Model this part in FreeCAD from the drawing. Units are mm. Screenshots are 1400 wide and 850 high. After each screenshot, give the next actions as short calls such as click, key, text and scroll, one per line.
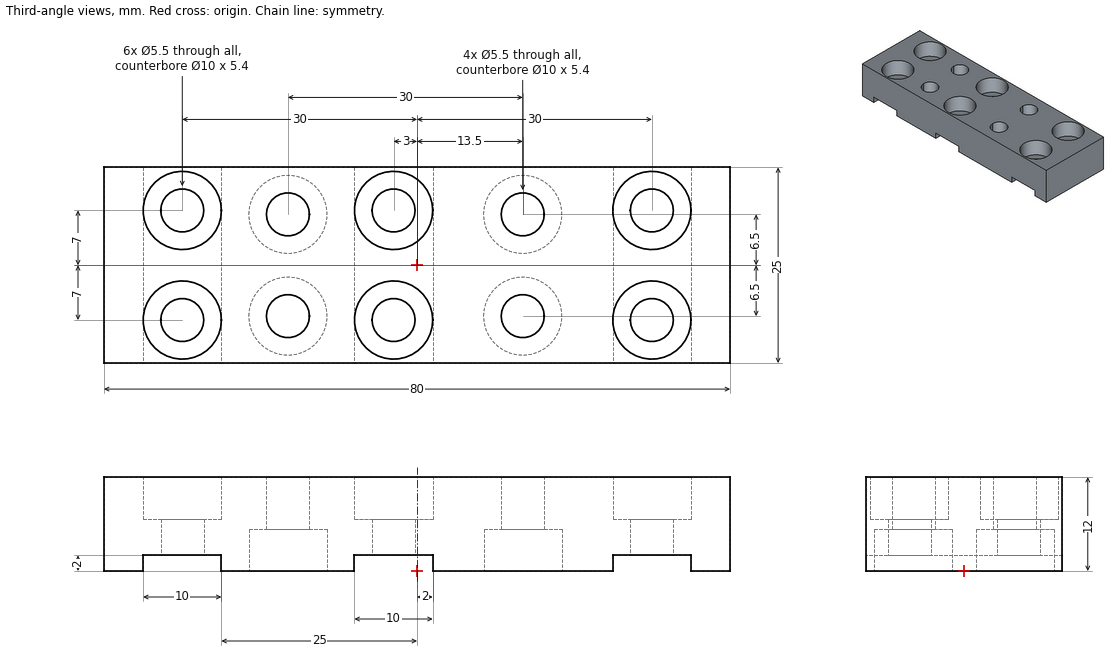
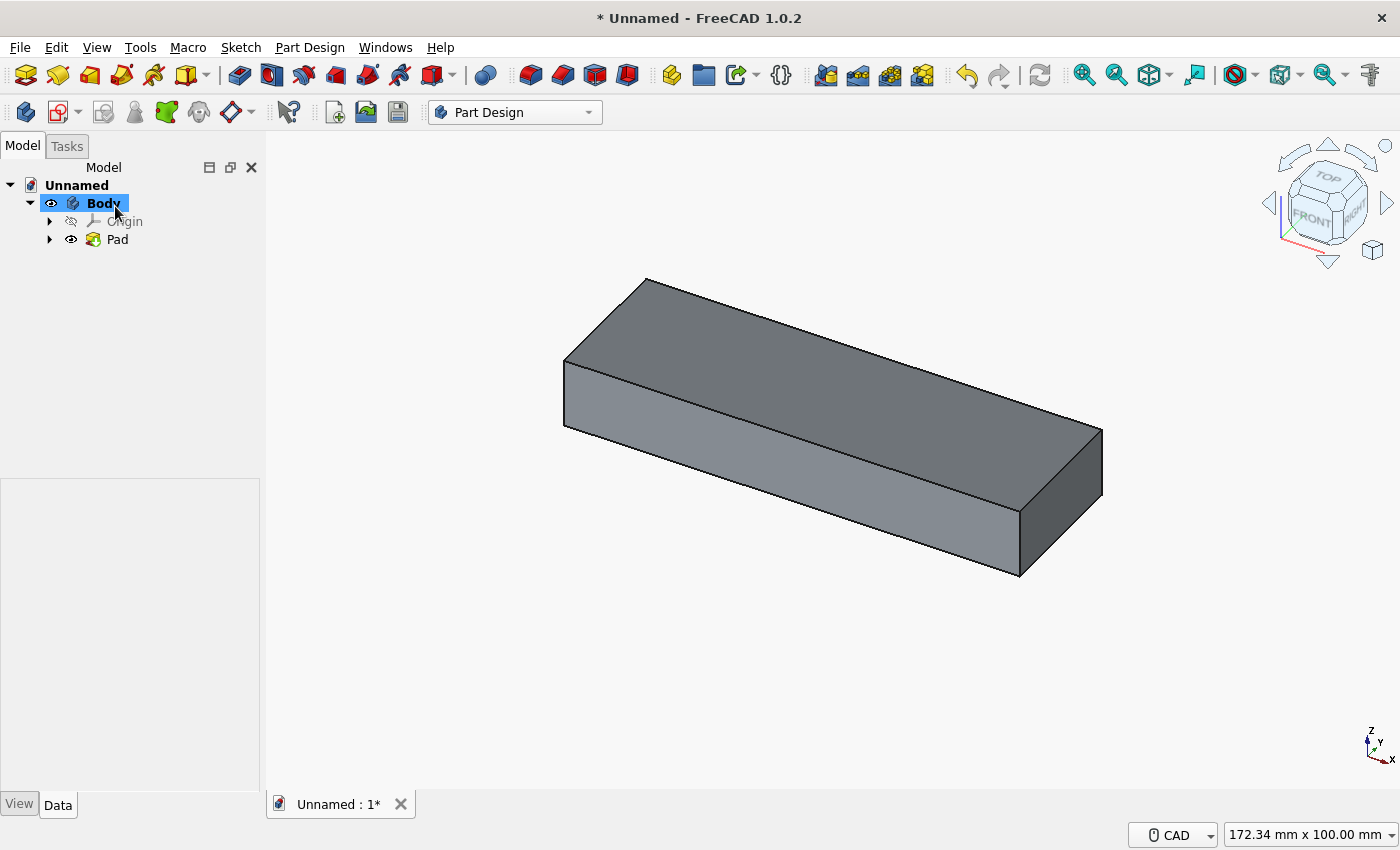
key(4)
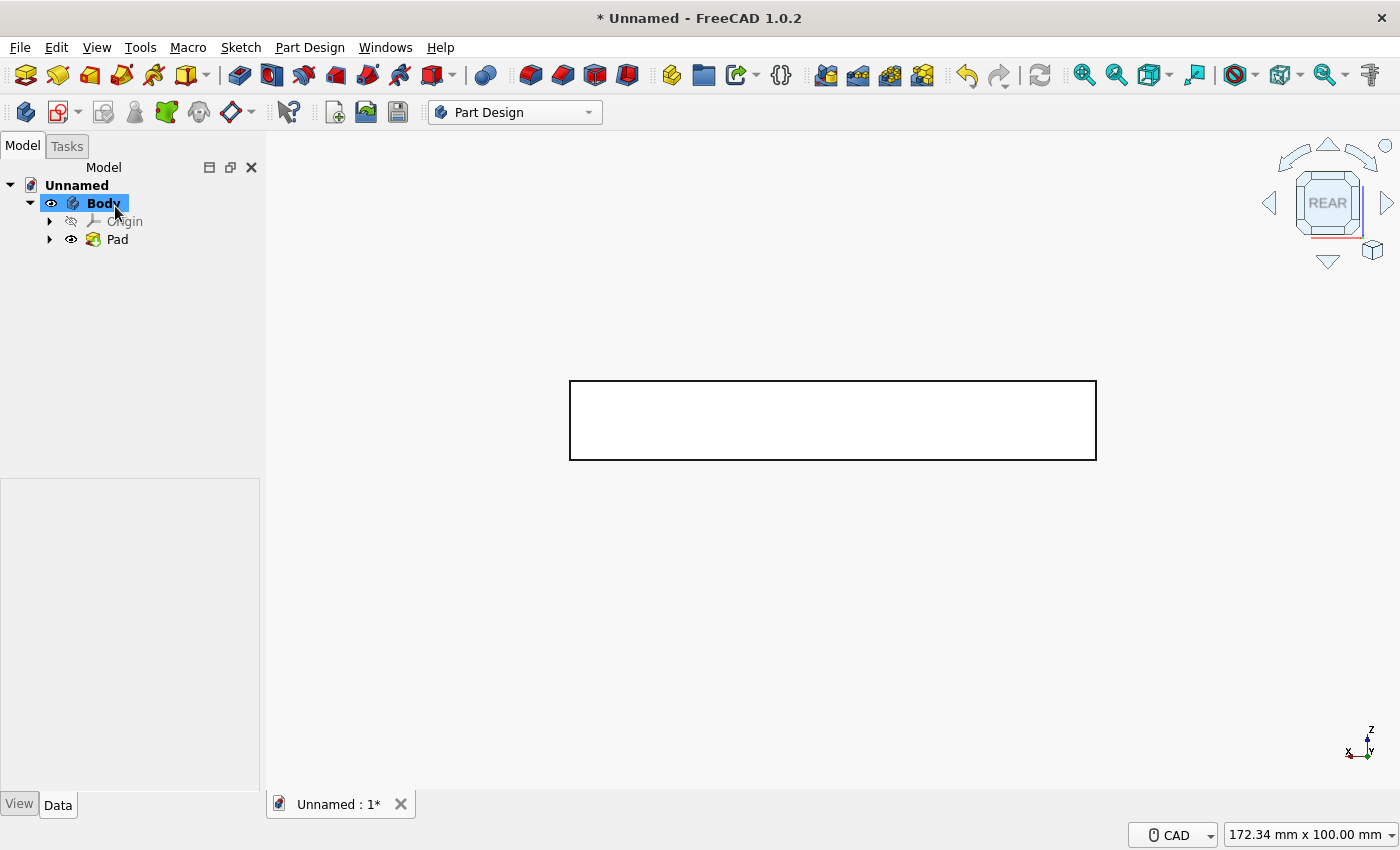
click(683, 420)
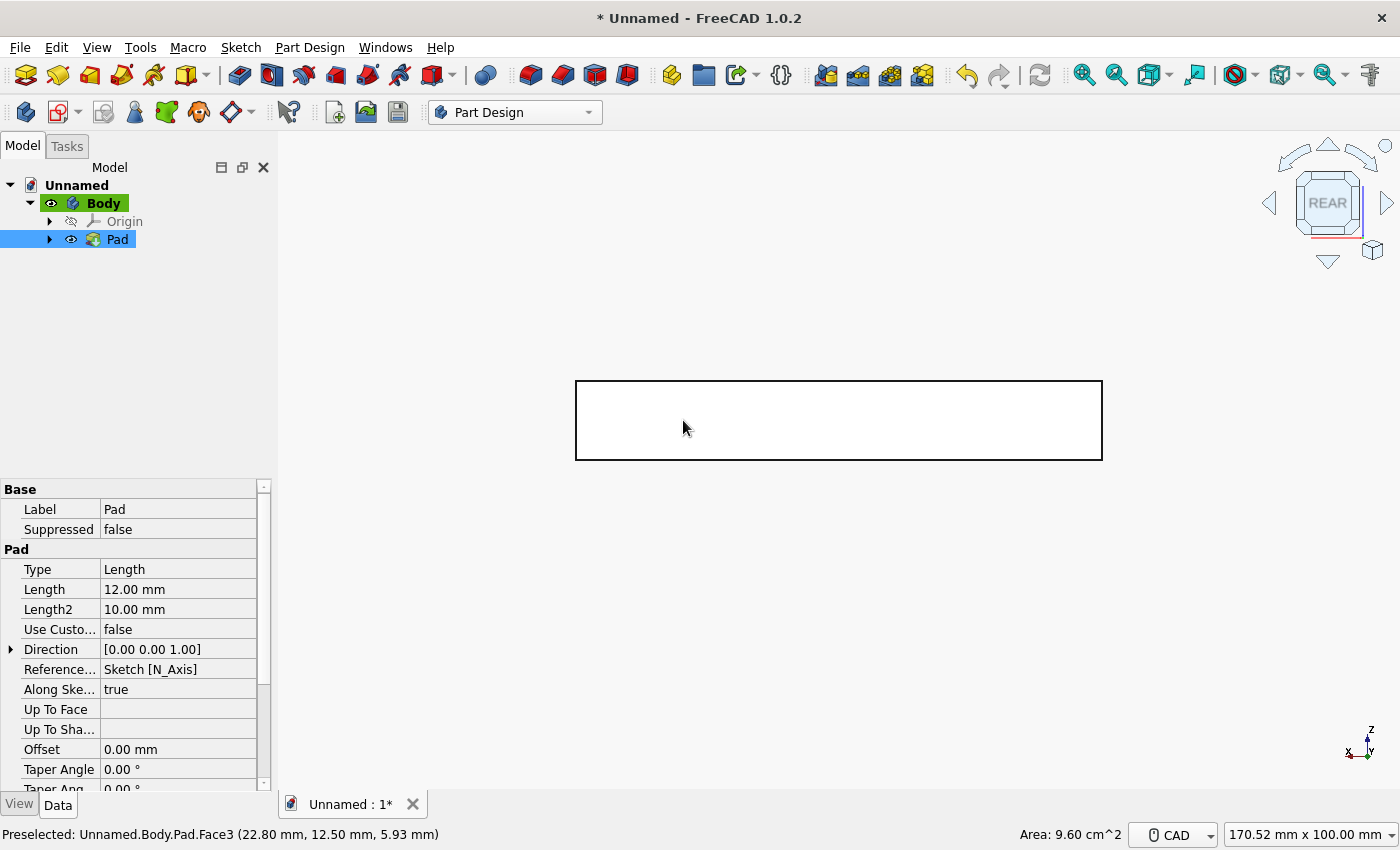
click(58, 112)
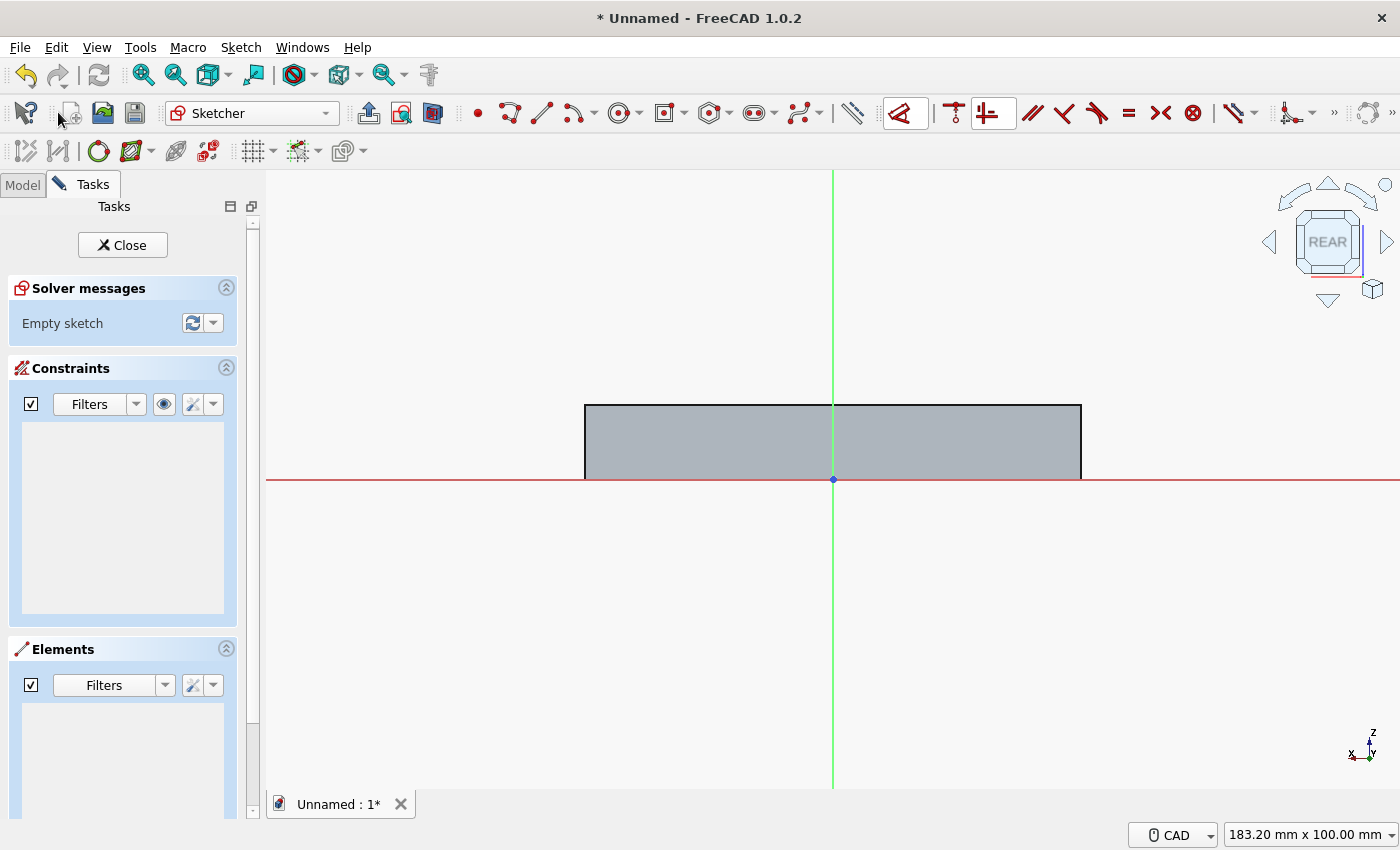
scroll(972, 461, up, 2)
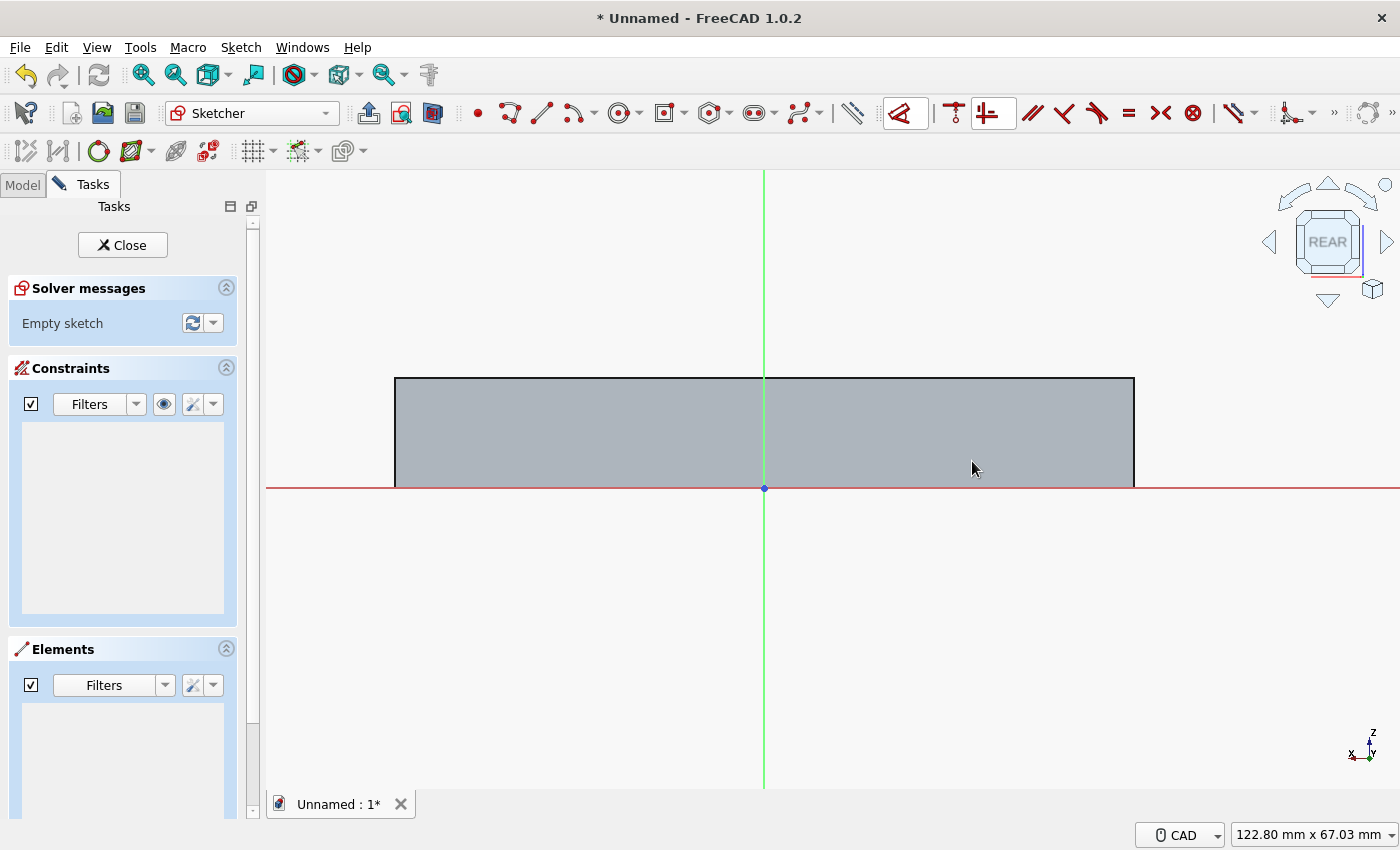
click(686, 114)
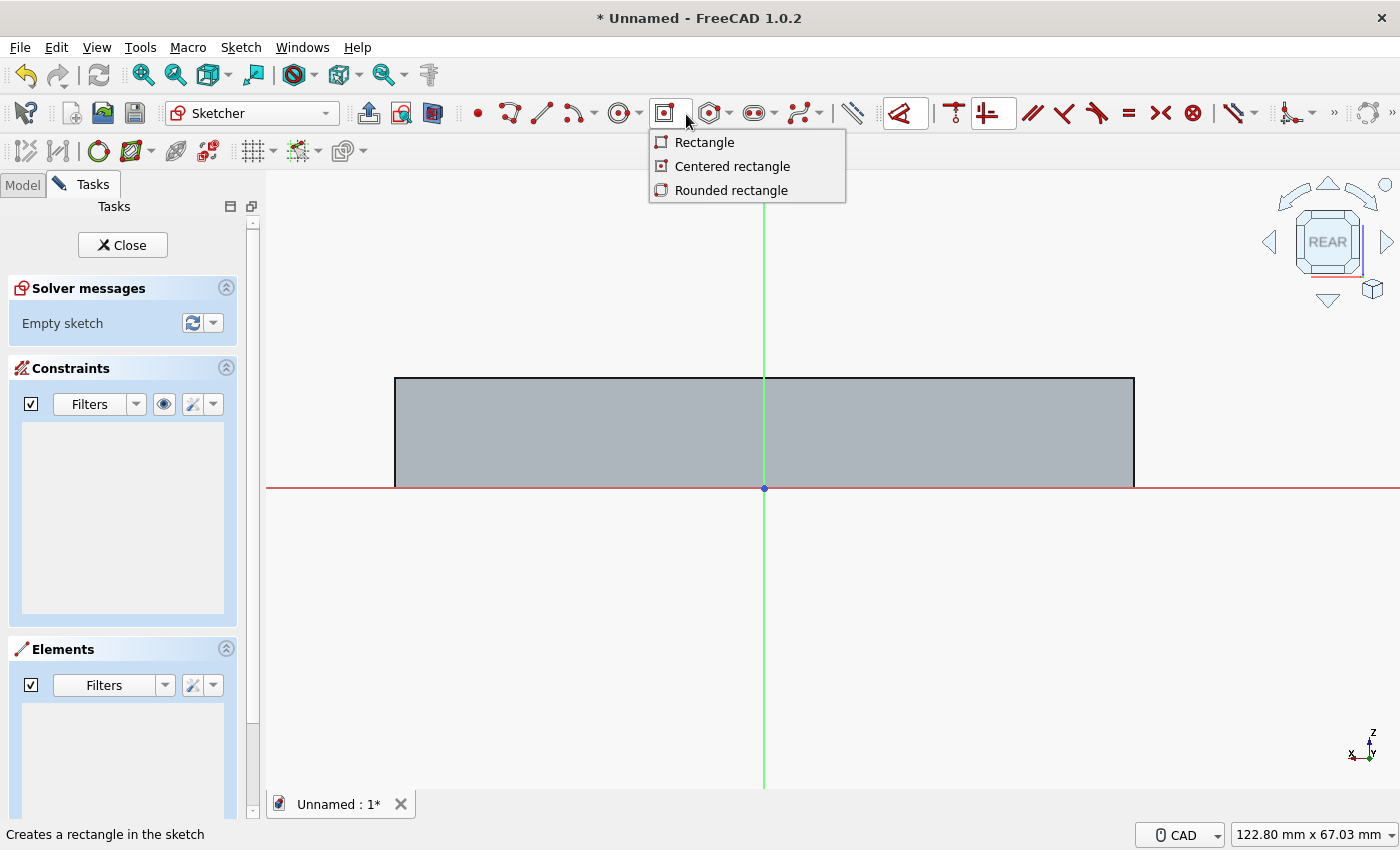
click(748, 142)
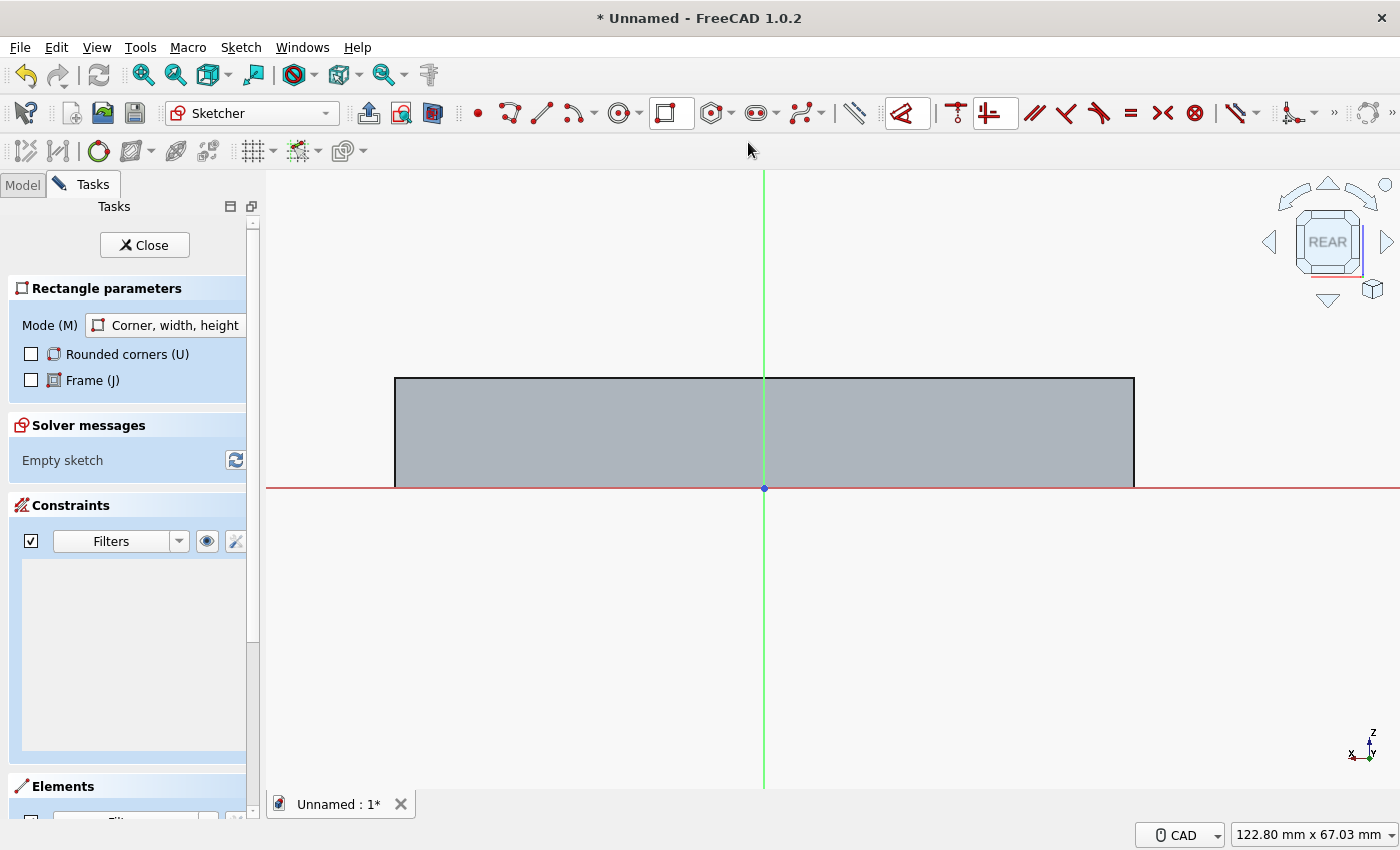
click(995, 470)
click(1088, 488)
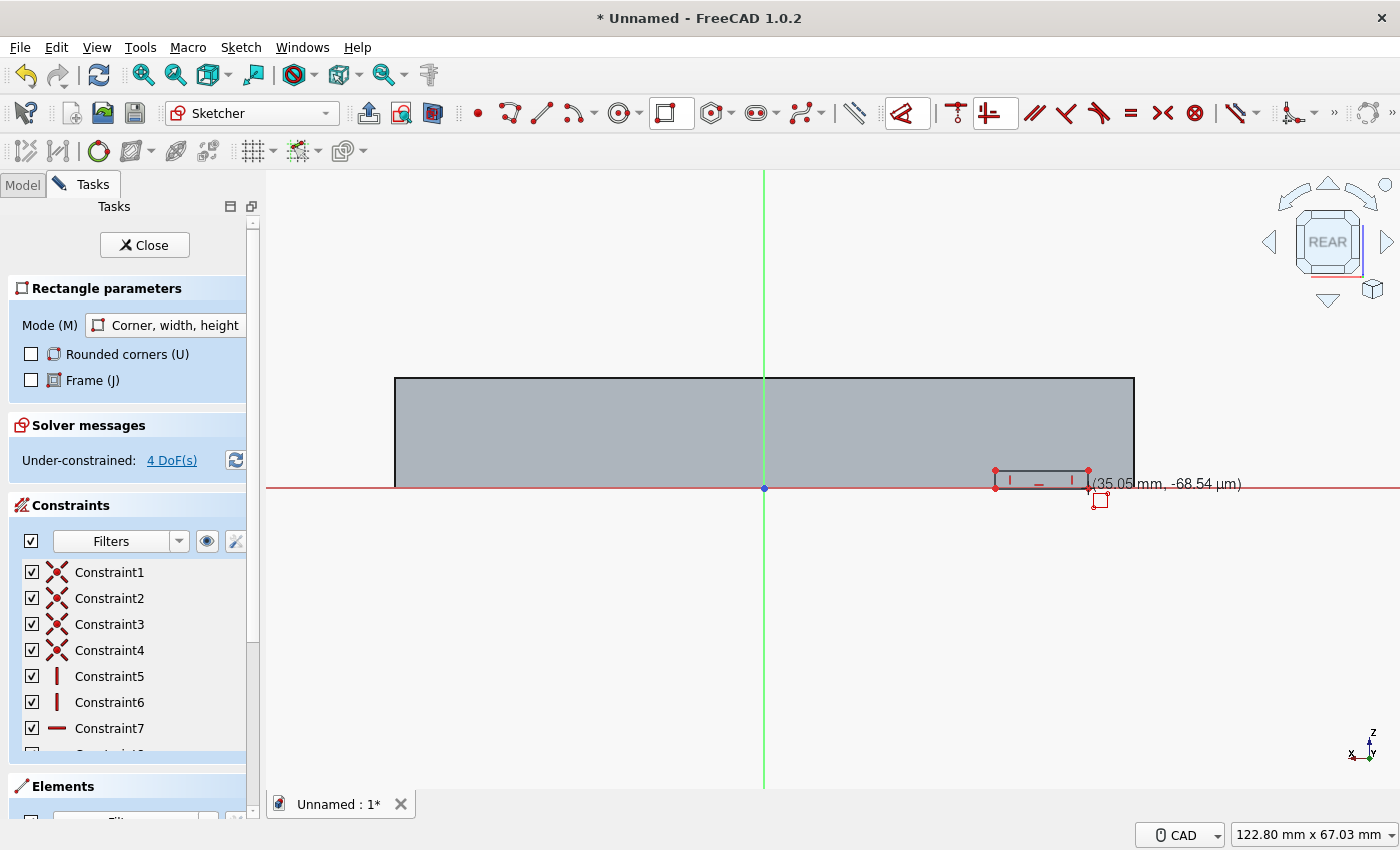
click(746, 470)
click(838, 488)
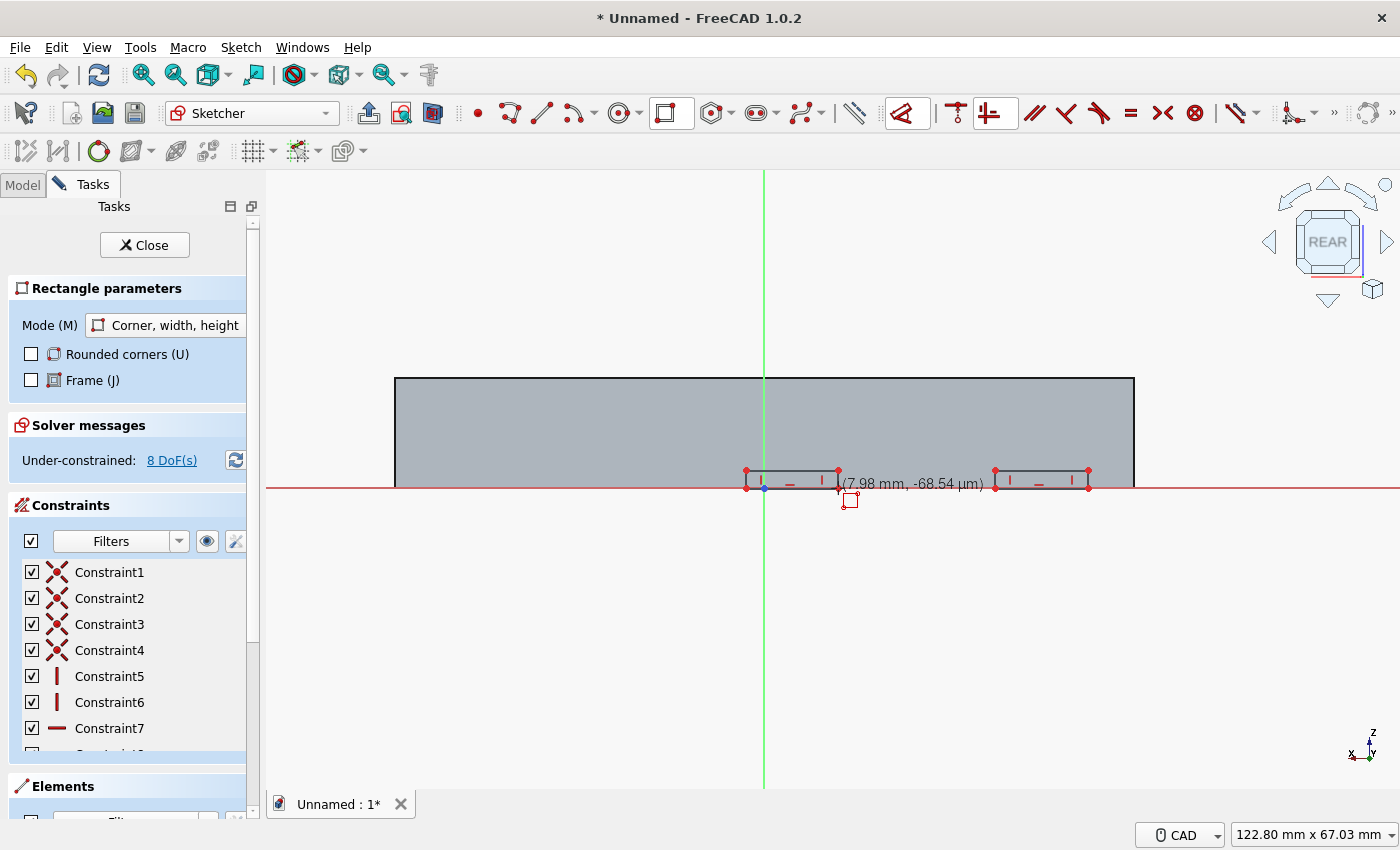
click(441, 470)
click(533, 488)
key(Escape)